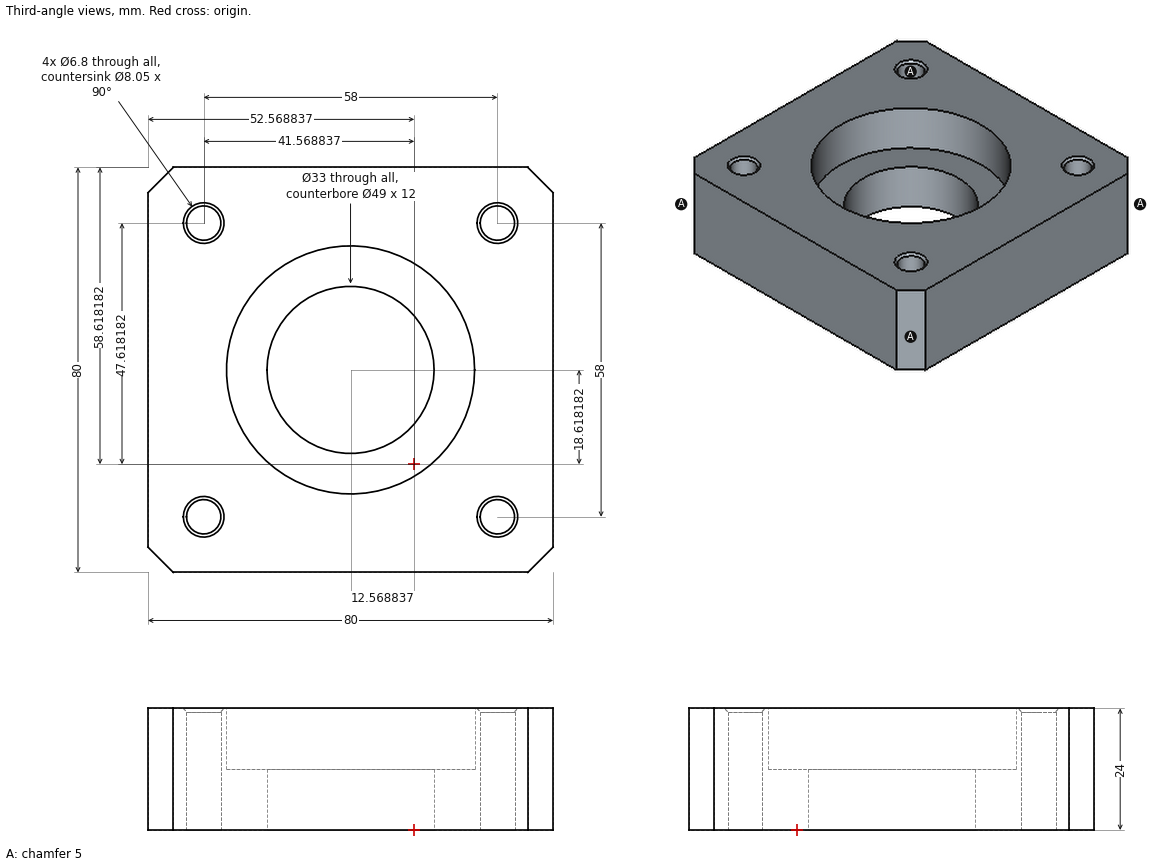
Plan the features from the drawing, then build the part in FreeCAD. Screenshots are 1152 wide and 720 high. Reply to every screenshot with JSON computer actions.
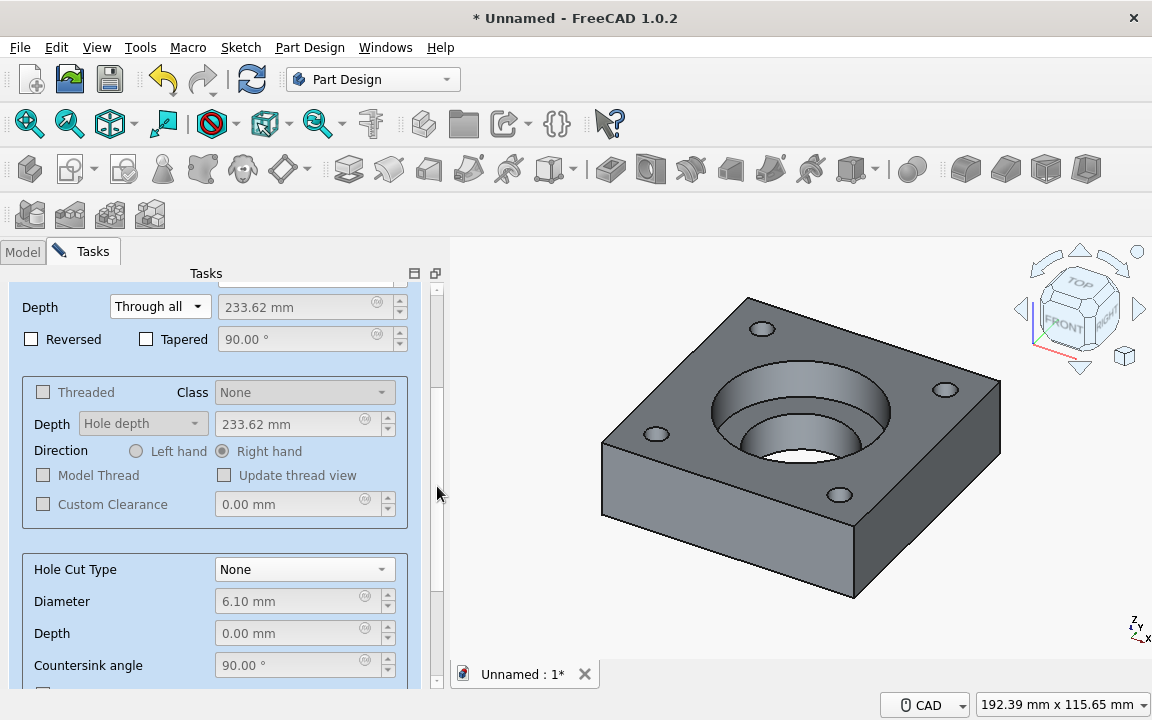
{"action": "left_click", "coordinate": [306, 570]}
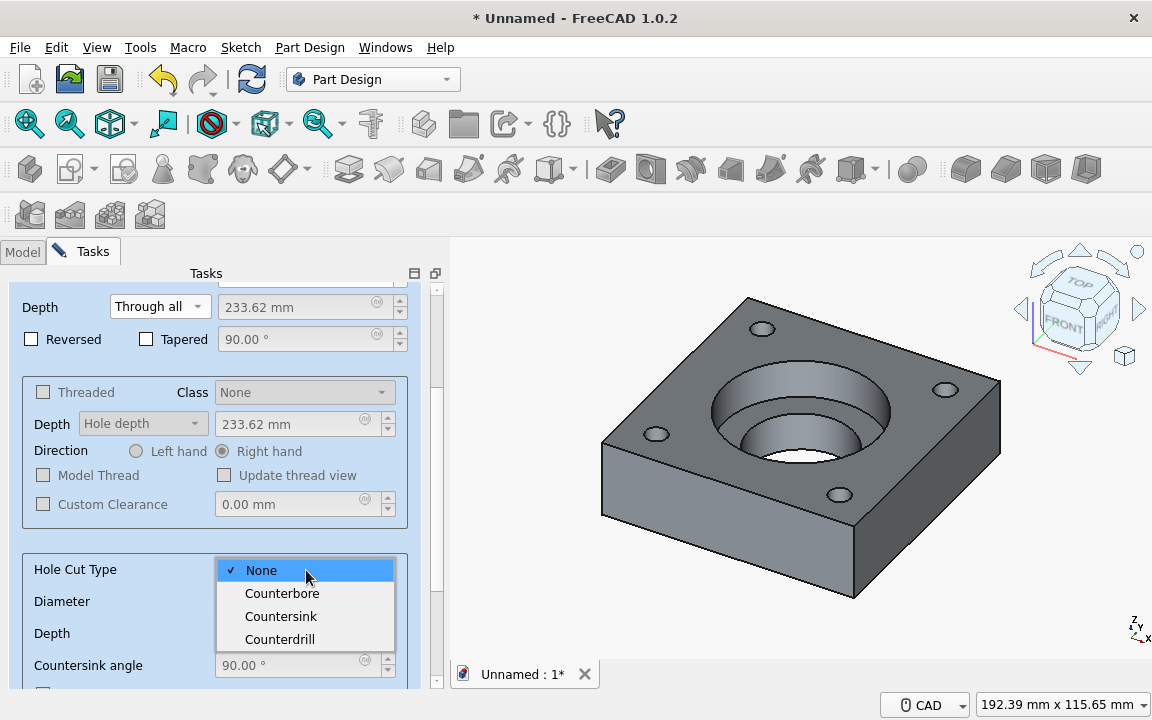
{"action": "left_click", "coordinate": [304, 616]}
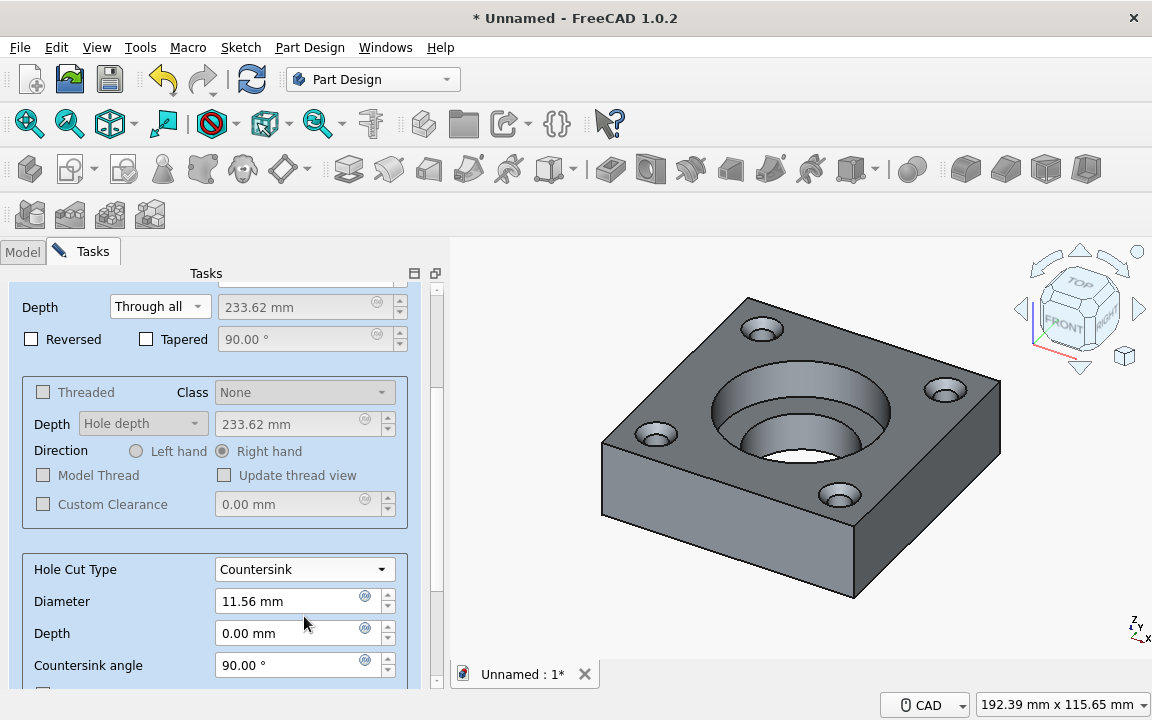
{"action": "triple_click", "coordinate": [298, 601]}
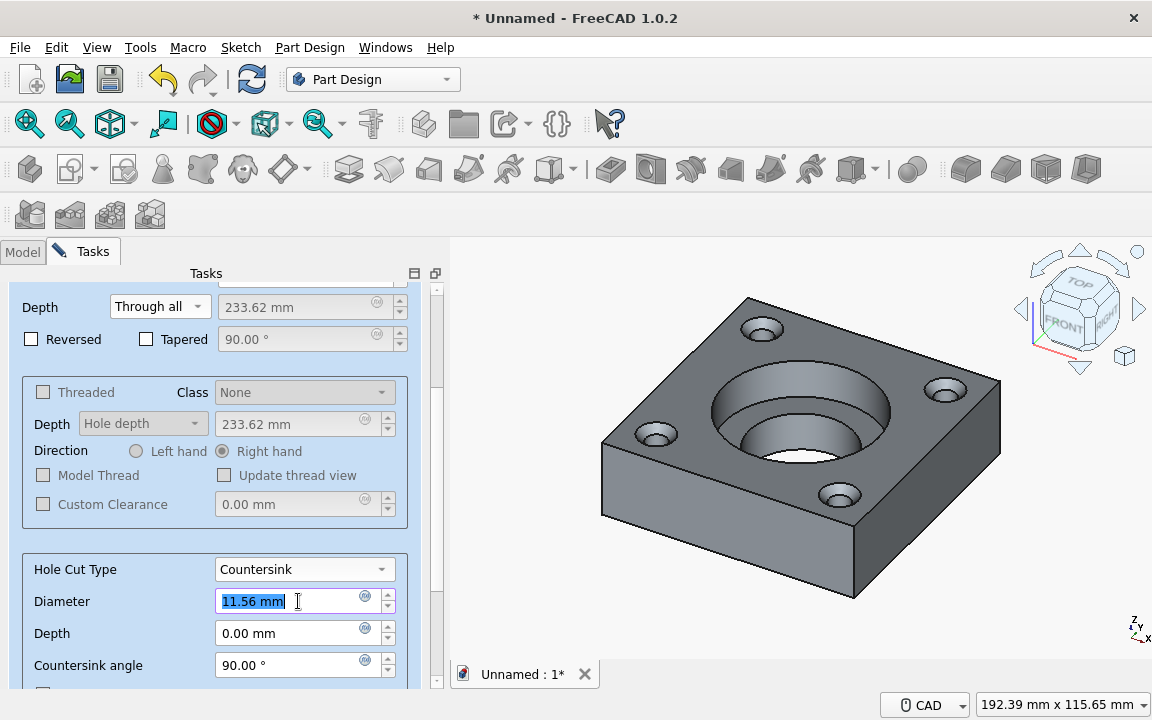
{"action": "type", "text": "8.05"}
{"action": "key", "text": "Tab"}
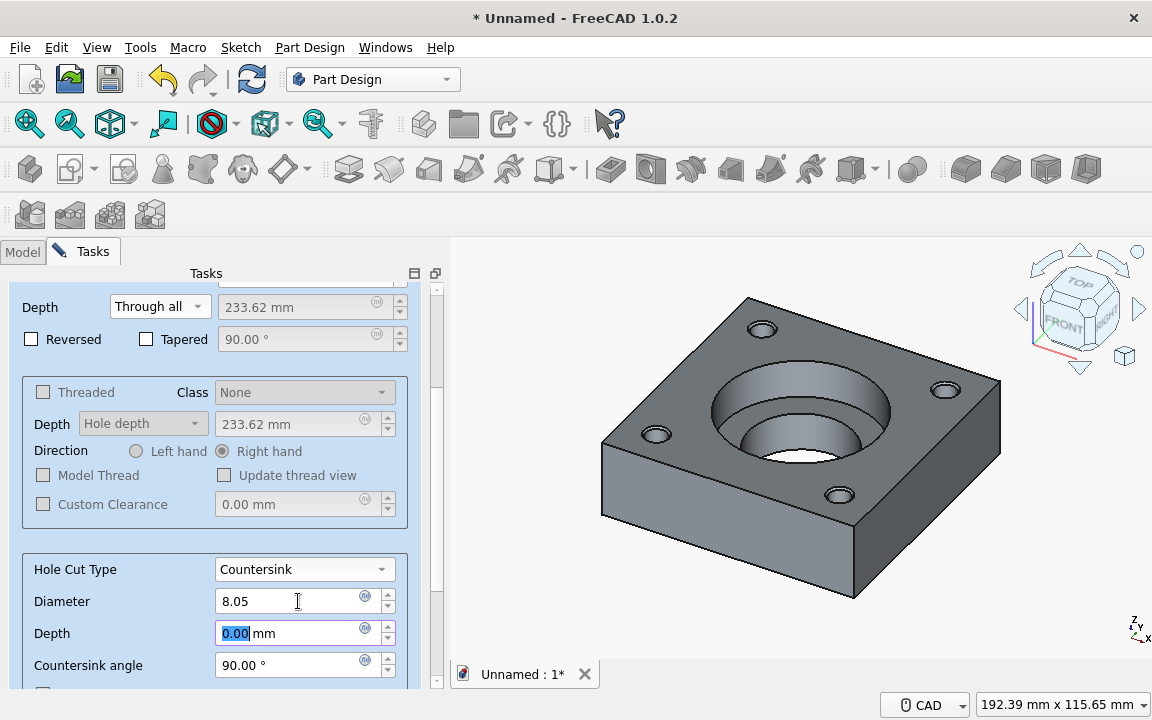
{"action": "scroll", "coordinate": [437, 486], "scroll_direction": "up", "scroll_amount": 4}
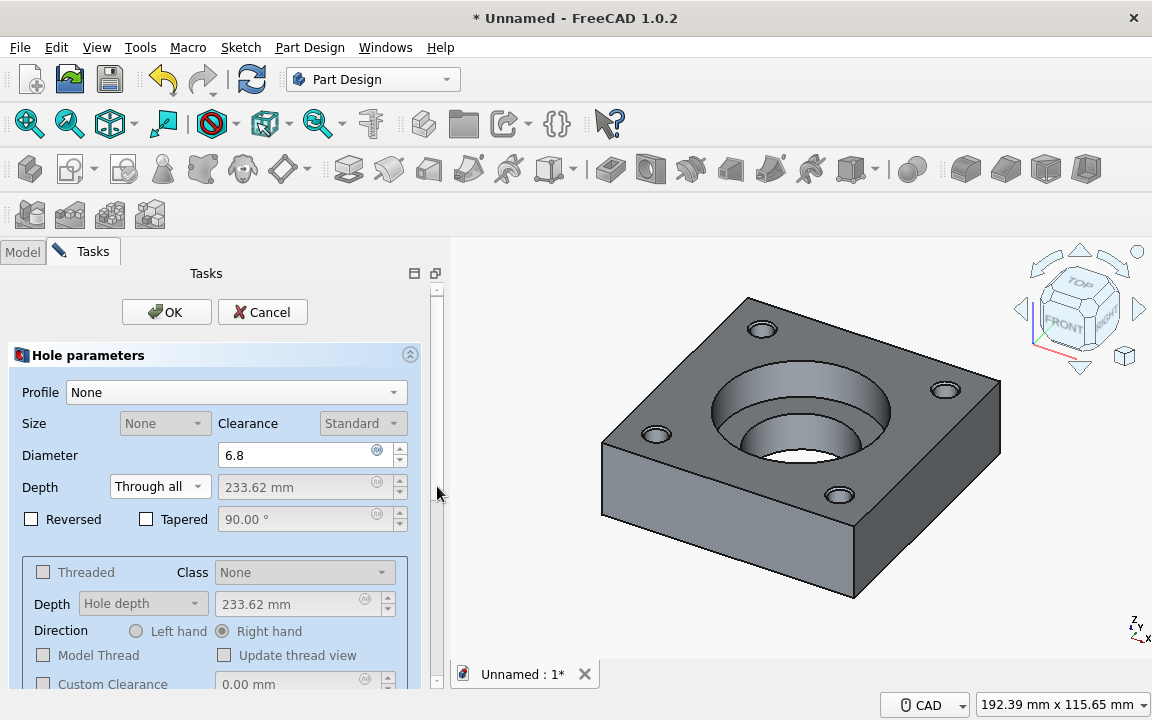
{"action": "left_click", "coordinate": [167, 312]}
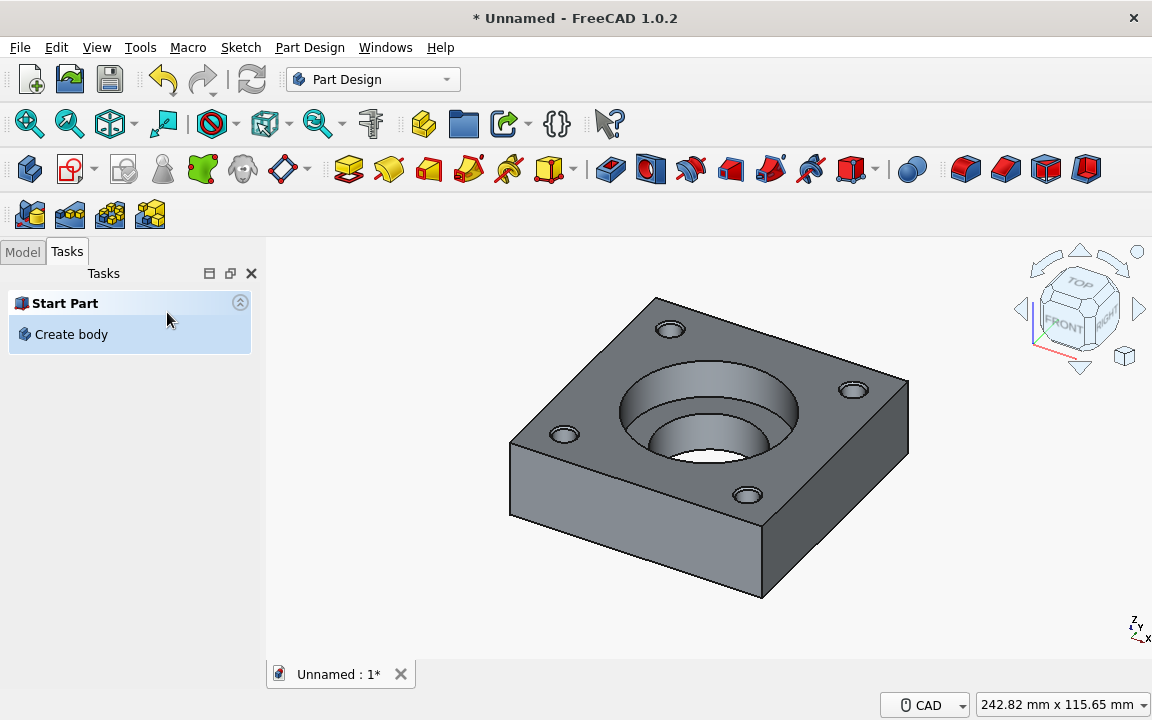
{"action": "left_click", "coordinate": [762, 561]}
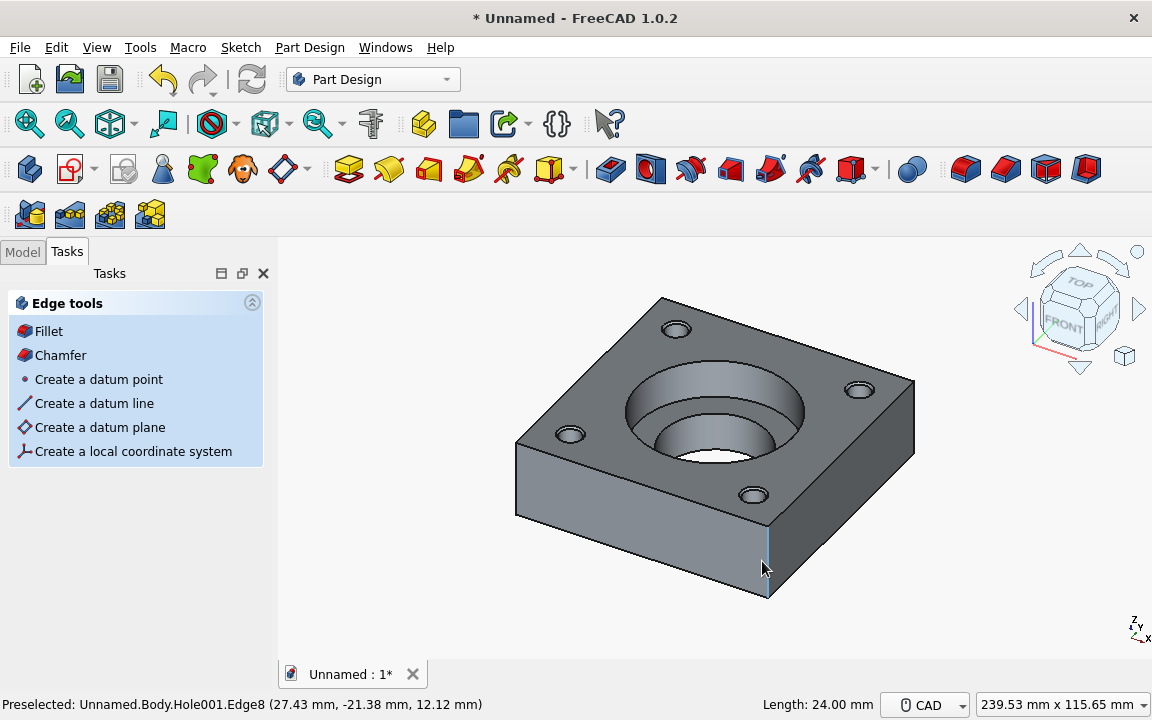
{"action": "key", "text": "0"}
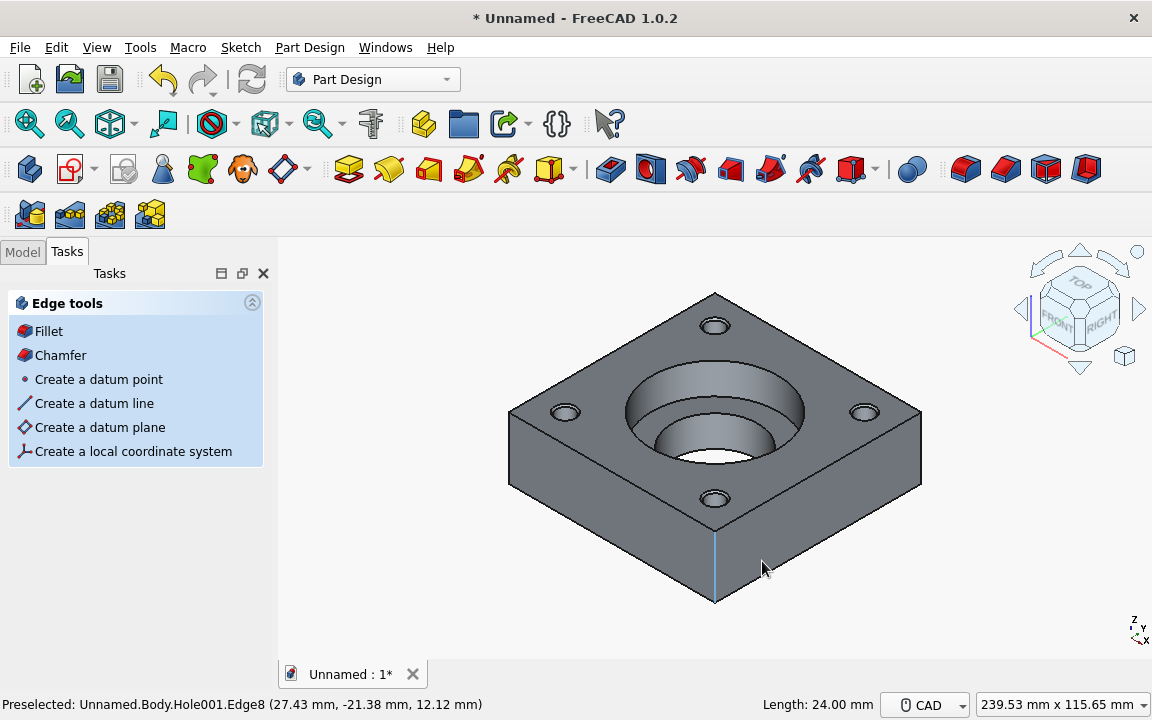
{"action": "key", "text": "2"}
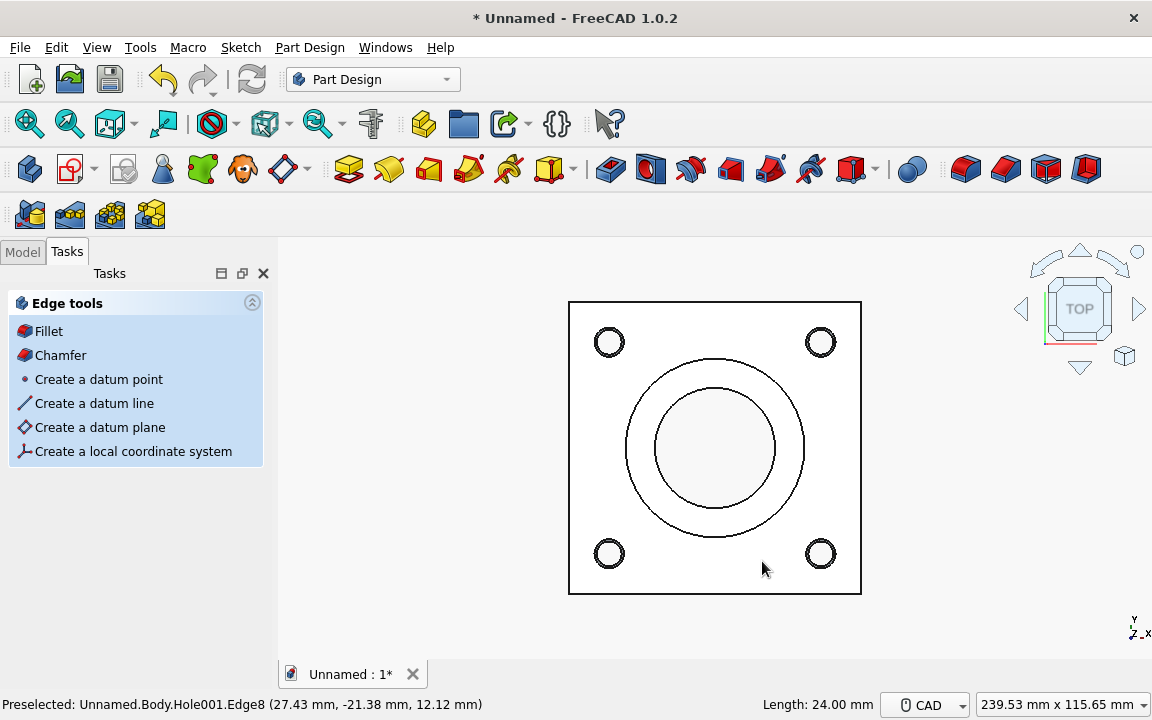
{"action": "key", "text": "1"}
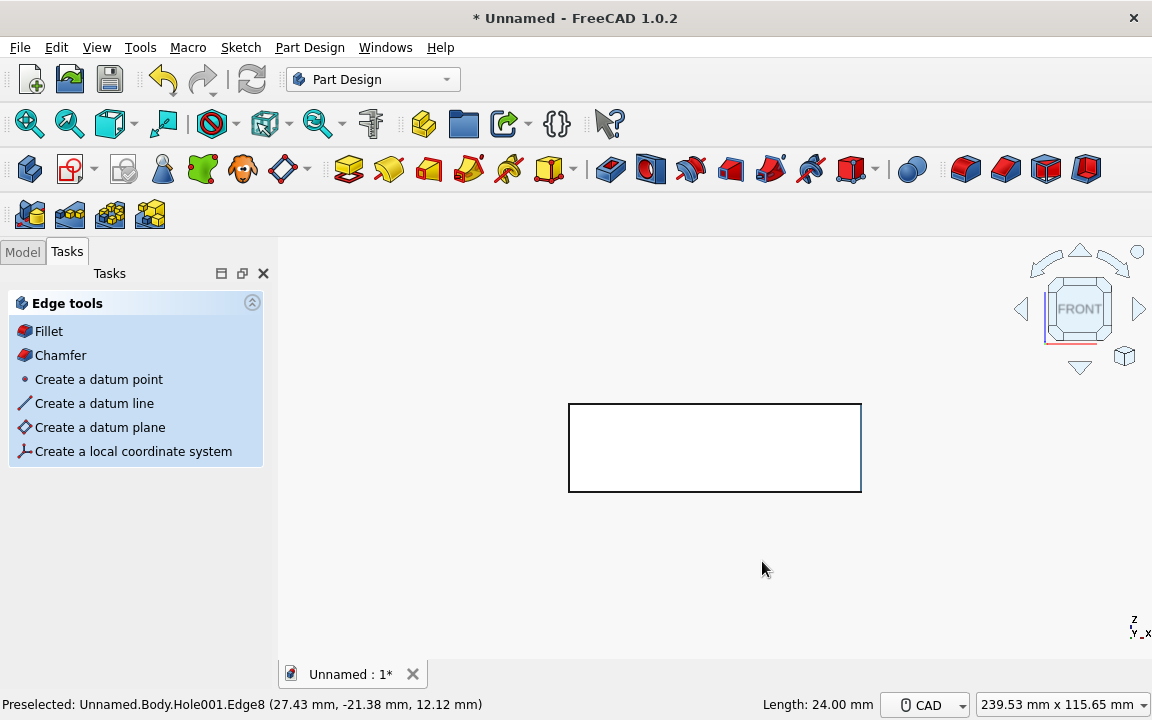
{"action": "left_click", "coordinate": [30, 124]}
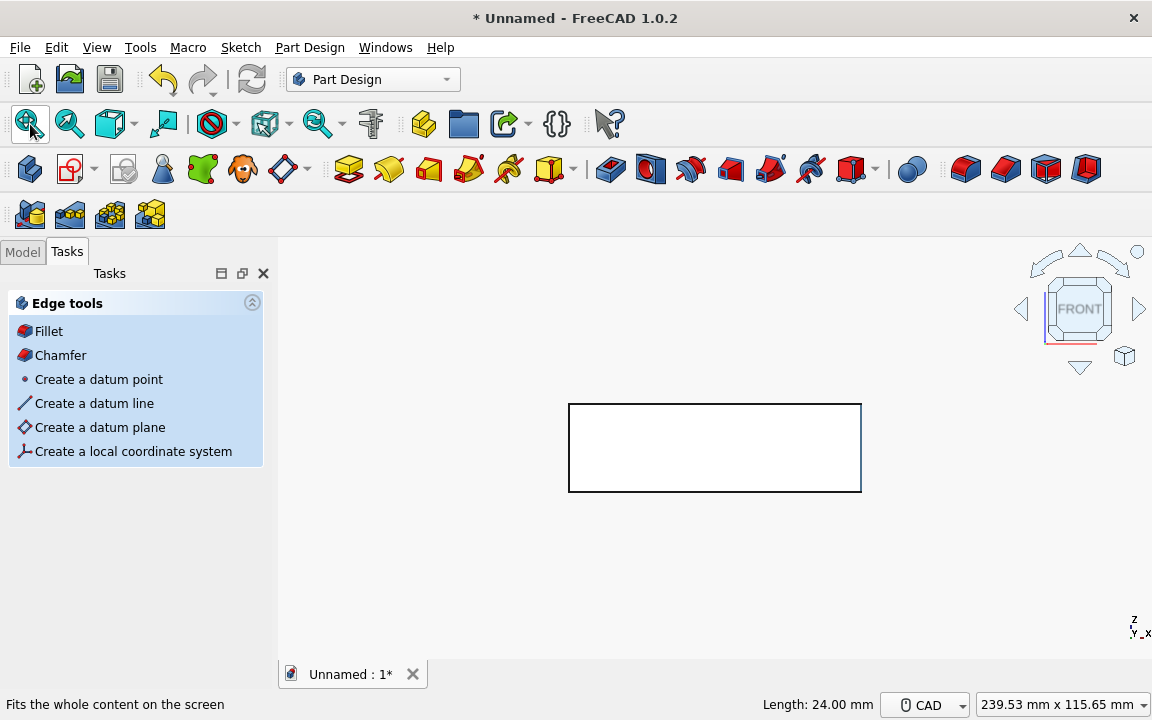
{"action": "left_click", "coordinate": [569, 447], "text": "ctrl"}